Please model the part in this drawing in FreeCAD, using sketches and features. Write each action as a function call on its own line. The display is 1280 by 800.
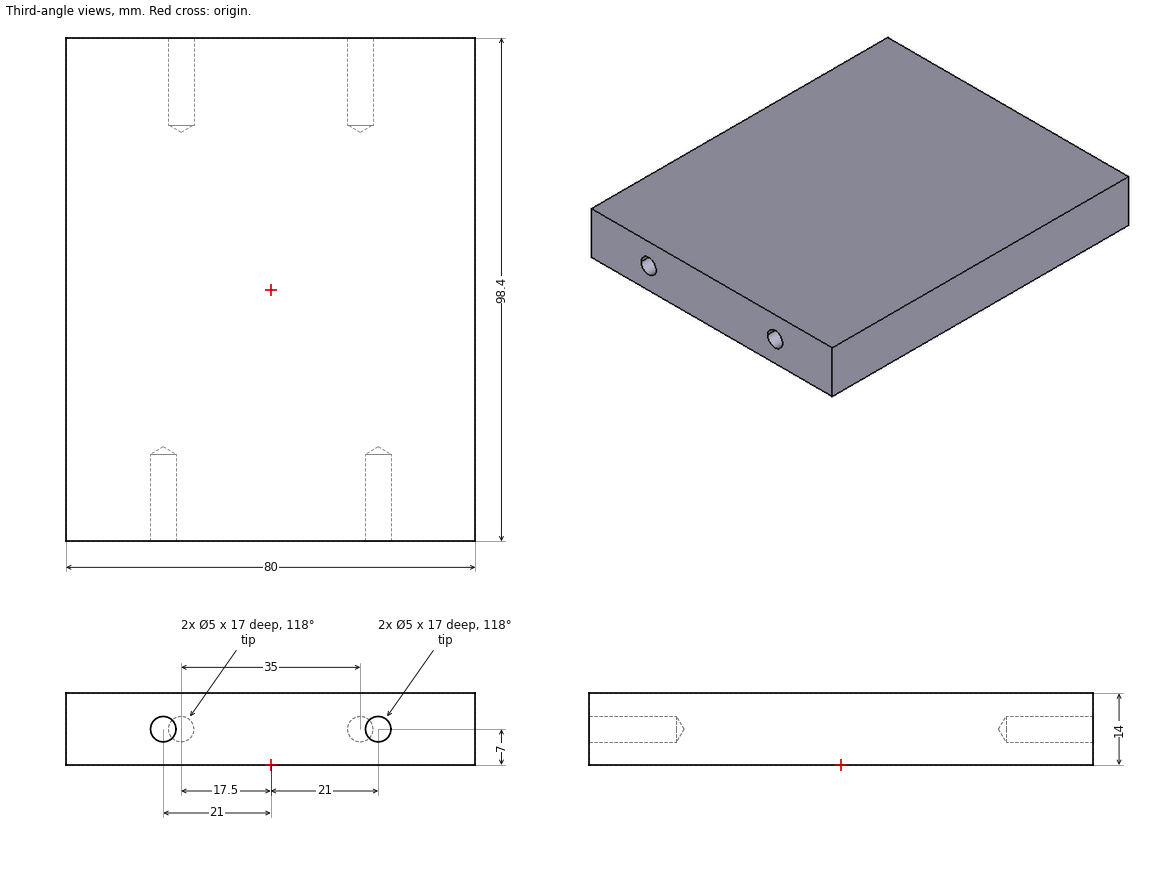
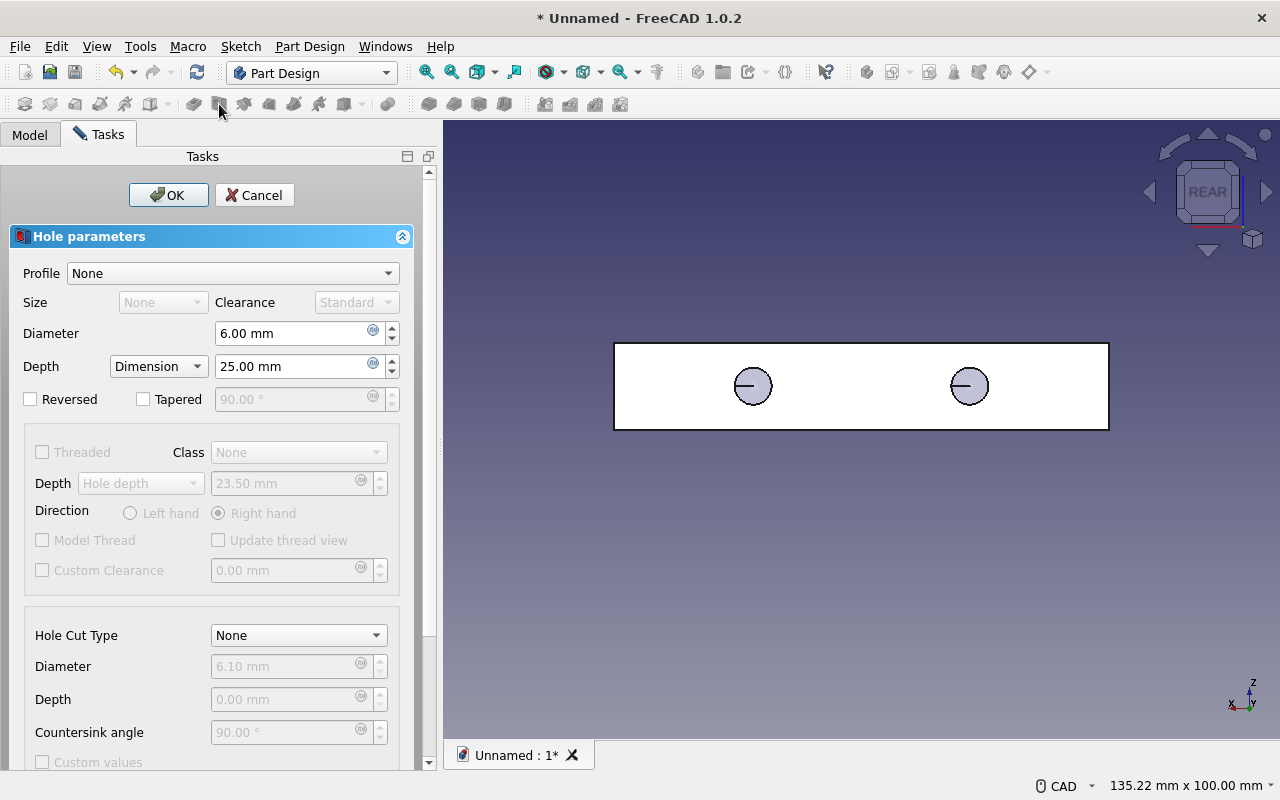
triple_click(300, 334)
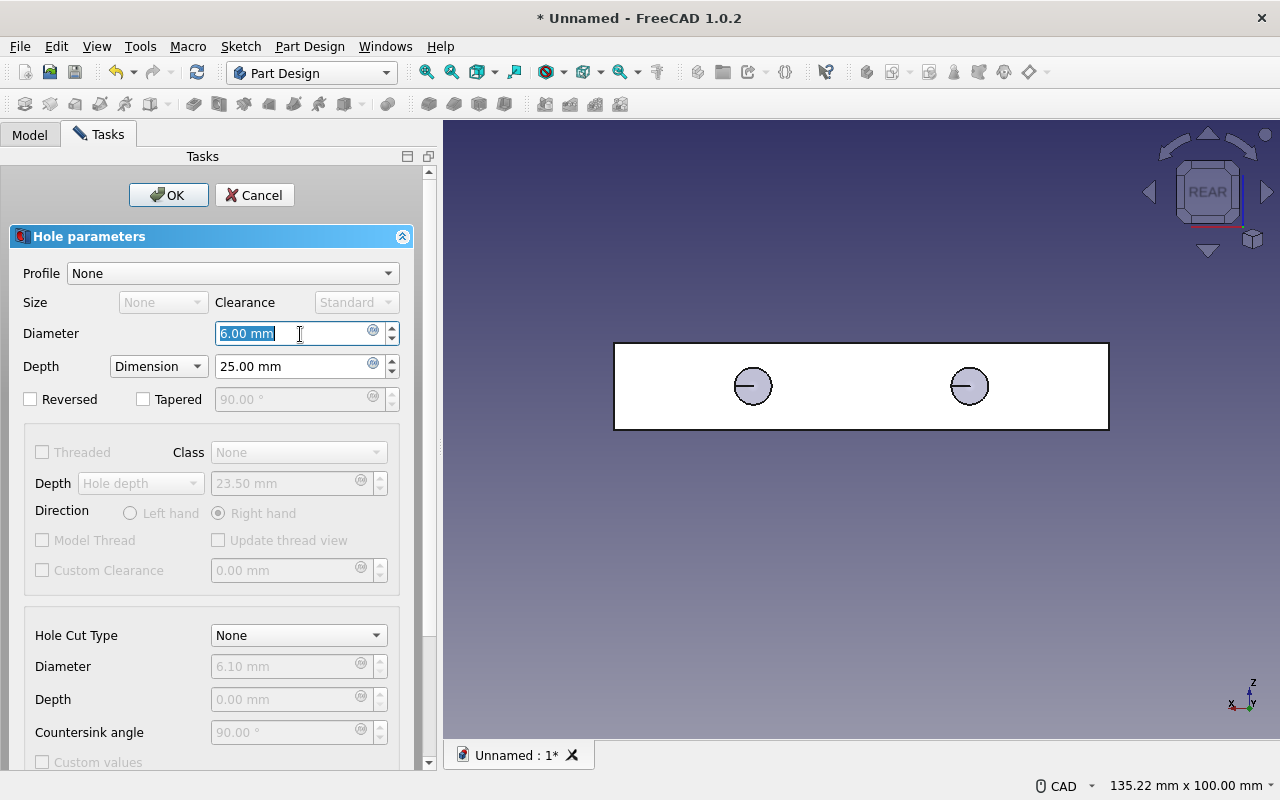
text(5)
key(Tab)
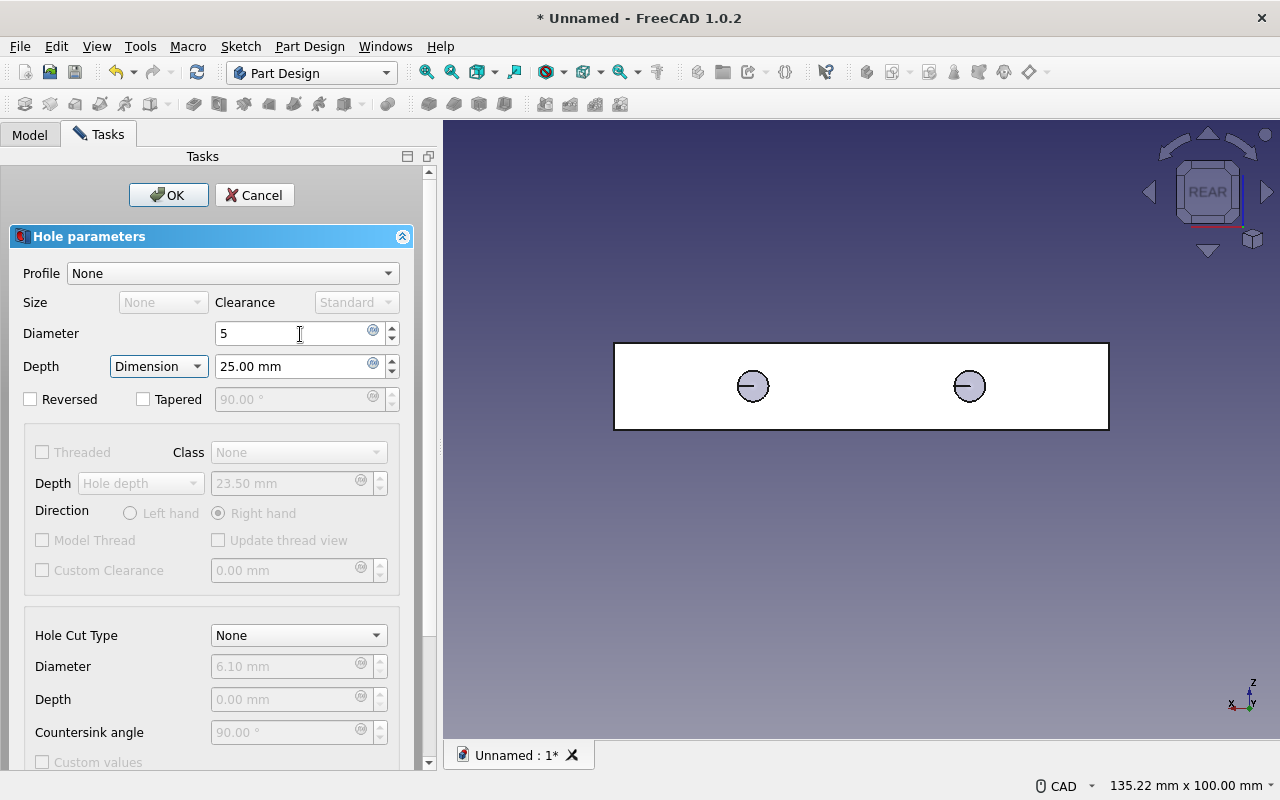
triple_click(300, 366)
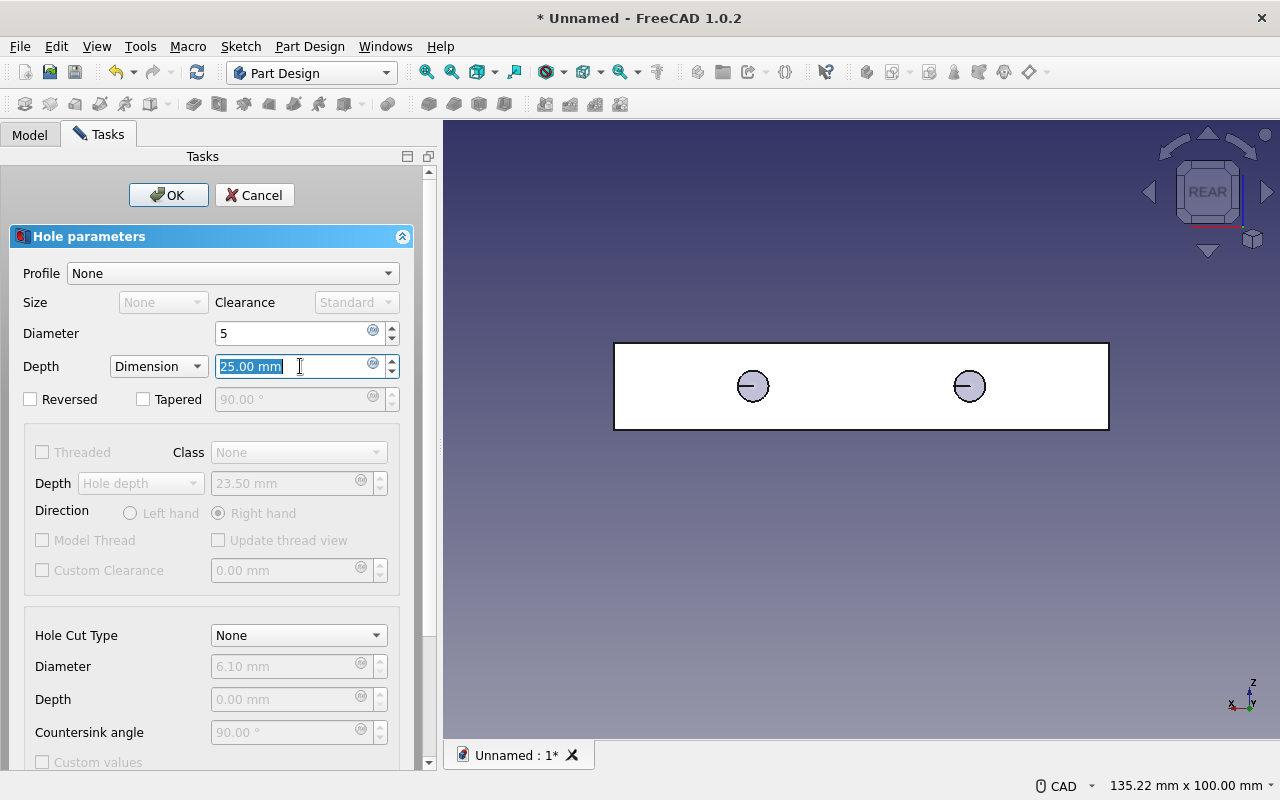
text(17)
key(Tab)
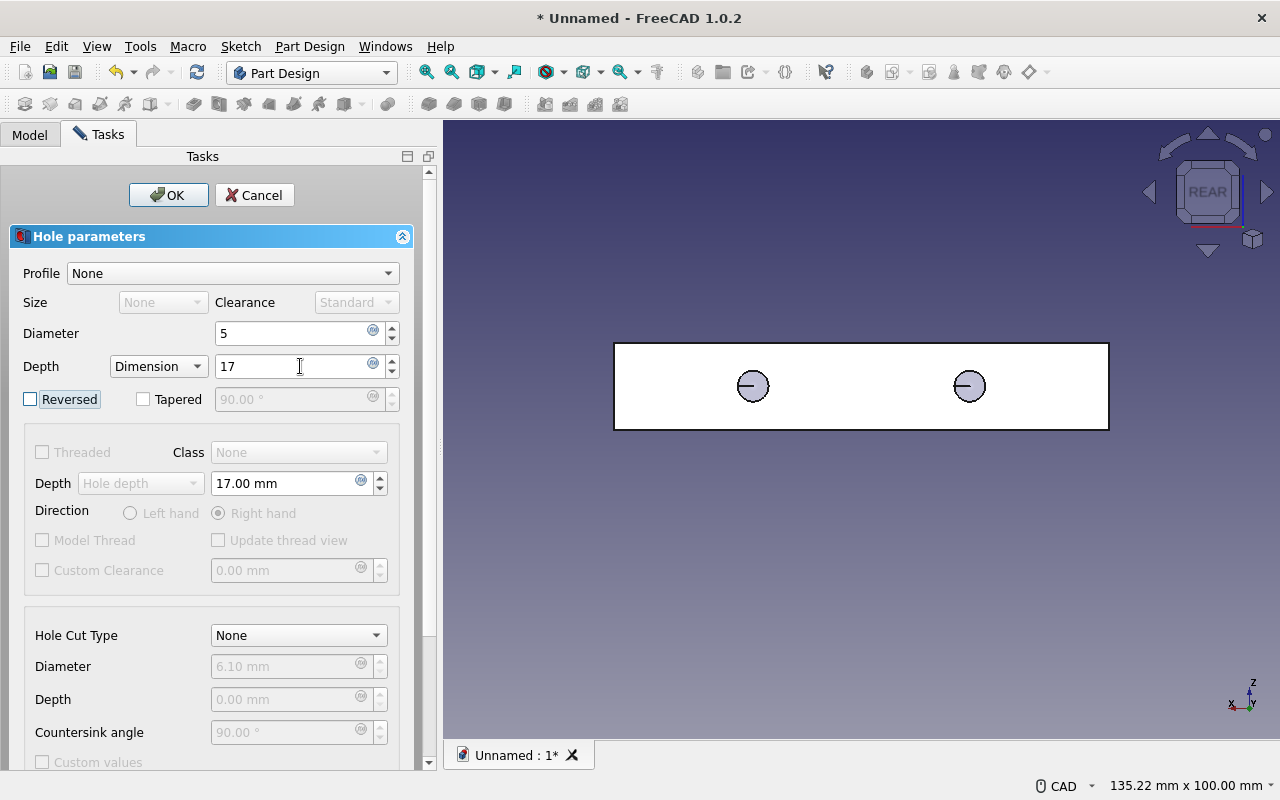
click(169, 195)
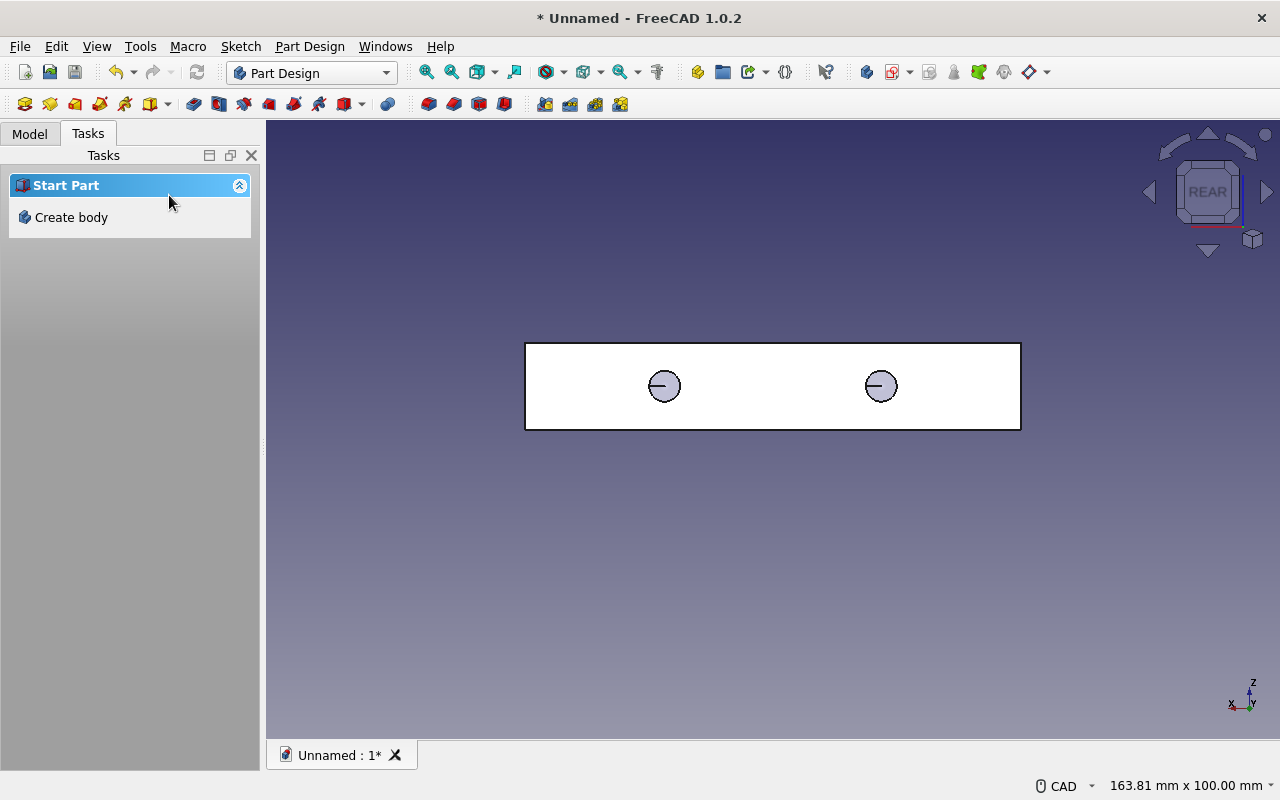
key(0)